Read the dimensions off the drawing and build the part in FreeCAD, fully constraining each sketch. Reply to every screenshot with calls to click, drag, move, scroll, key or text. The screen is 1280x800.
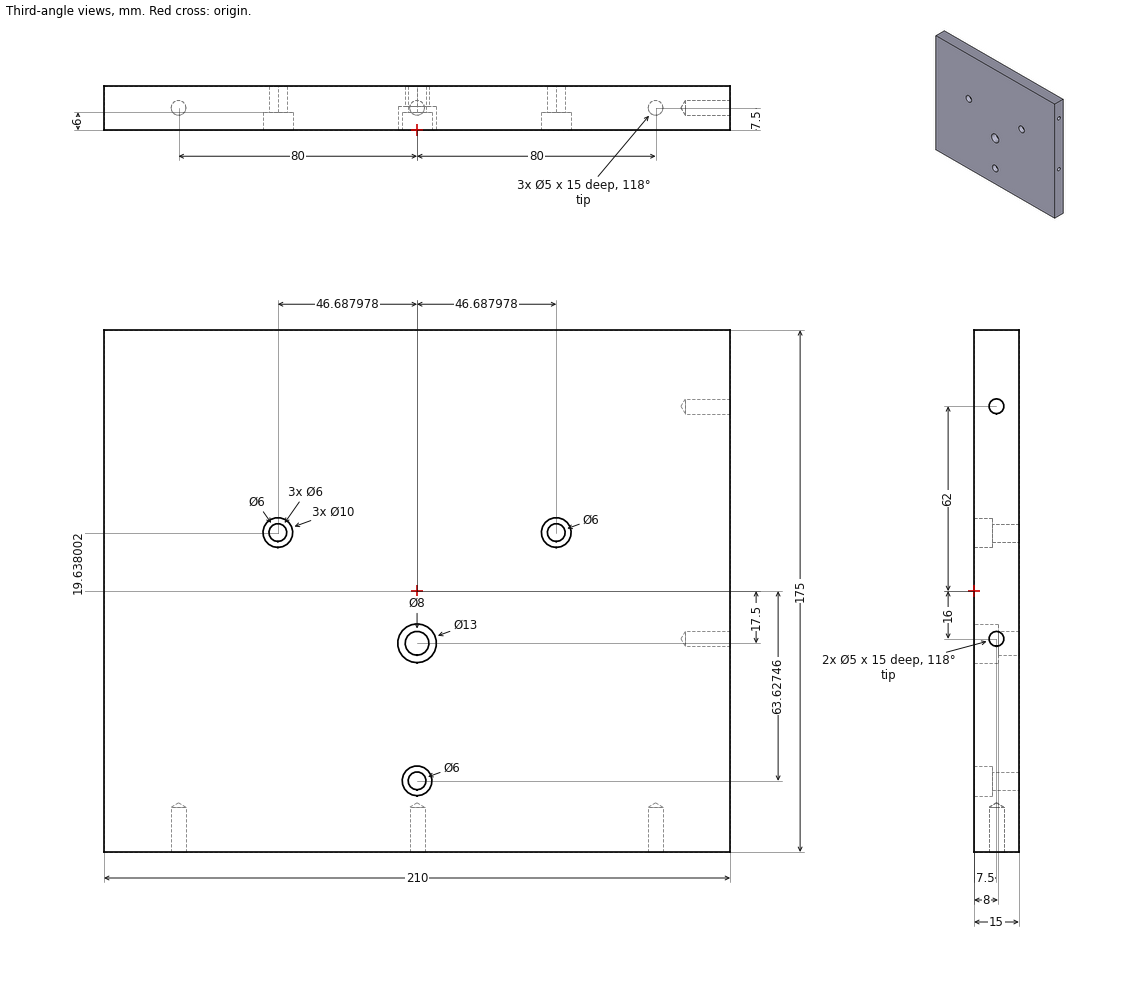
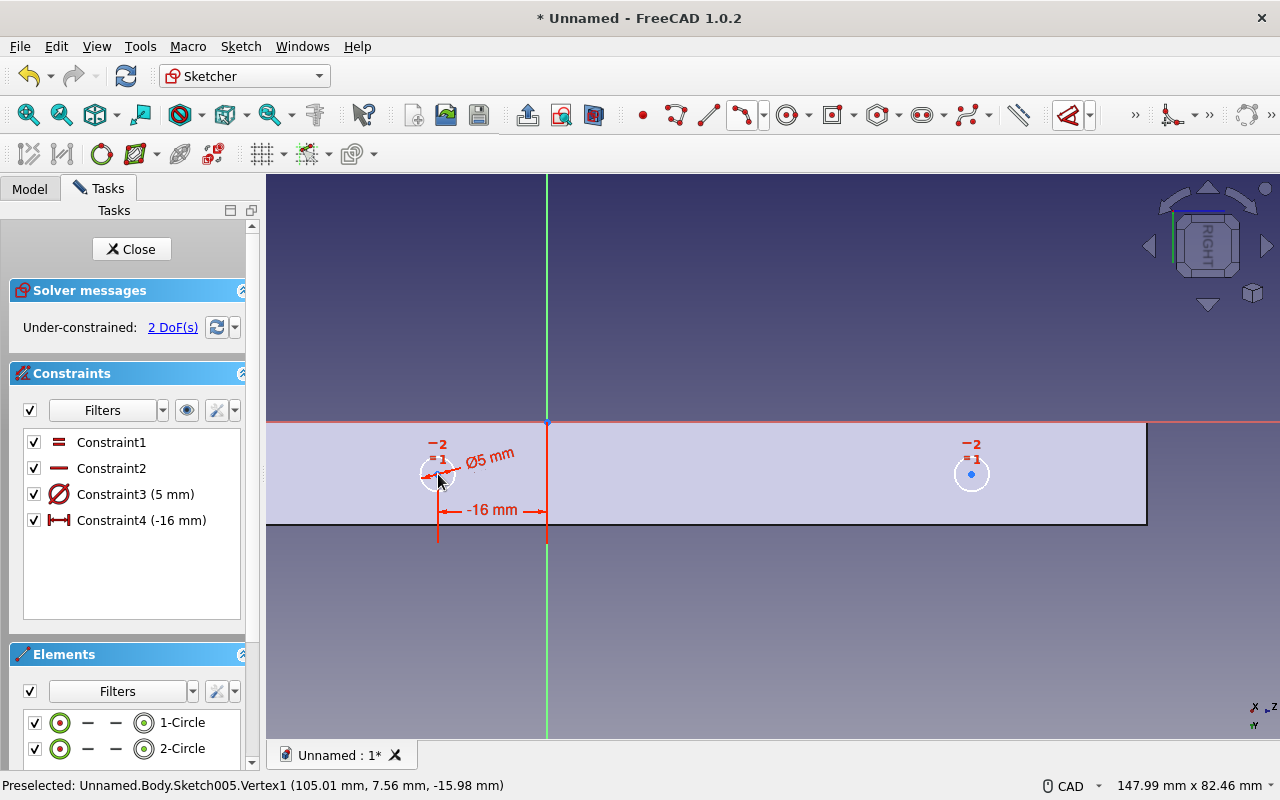
click(972, 474)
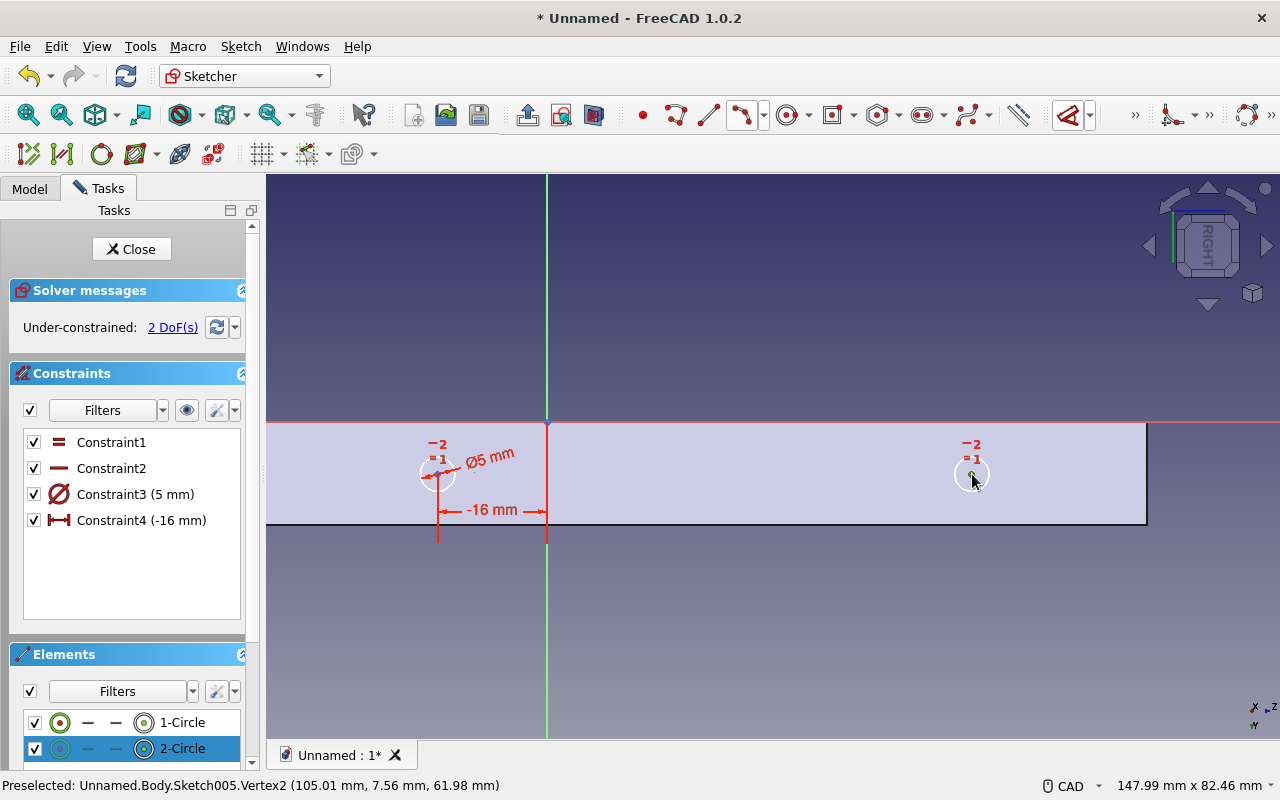
click(1090, 116)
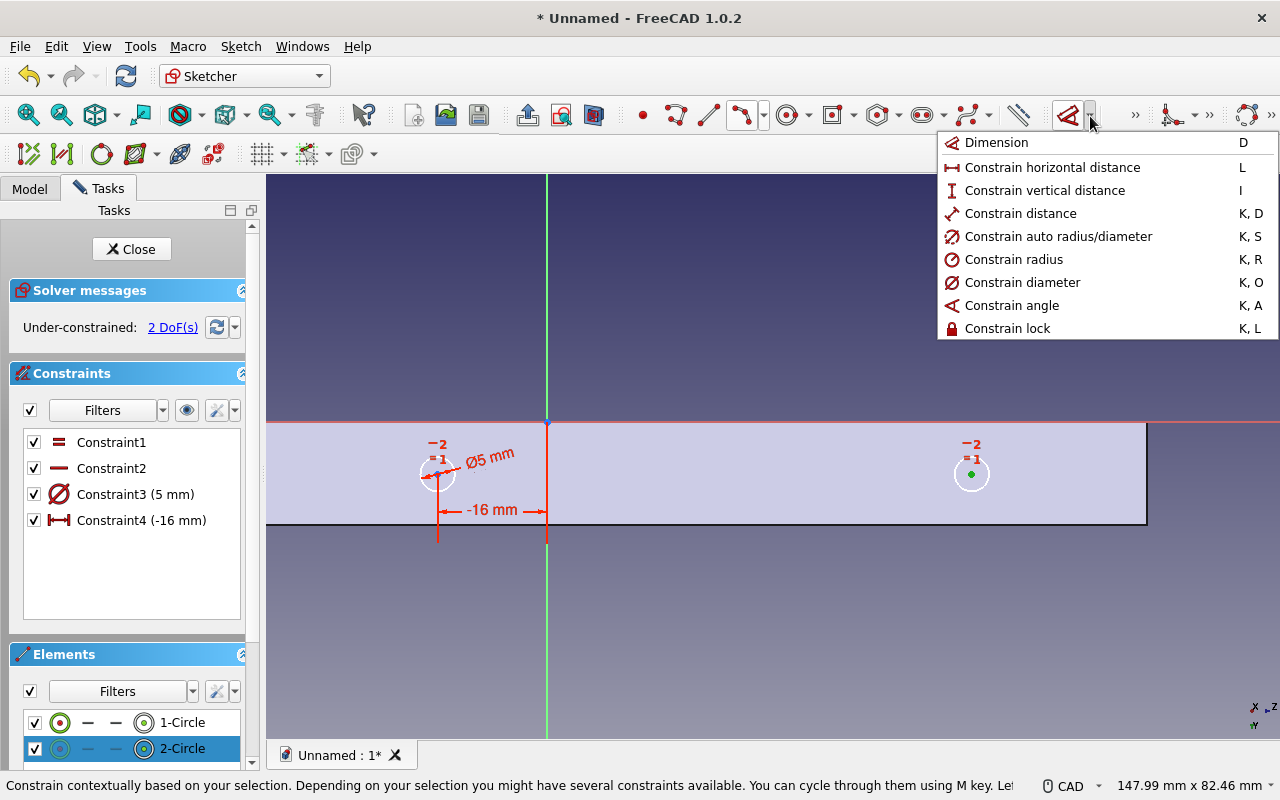
click(1108, 168)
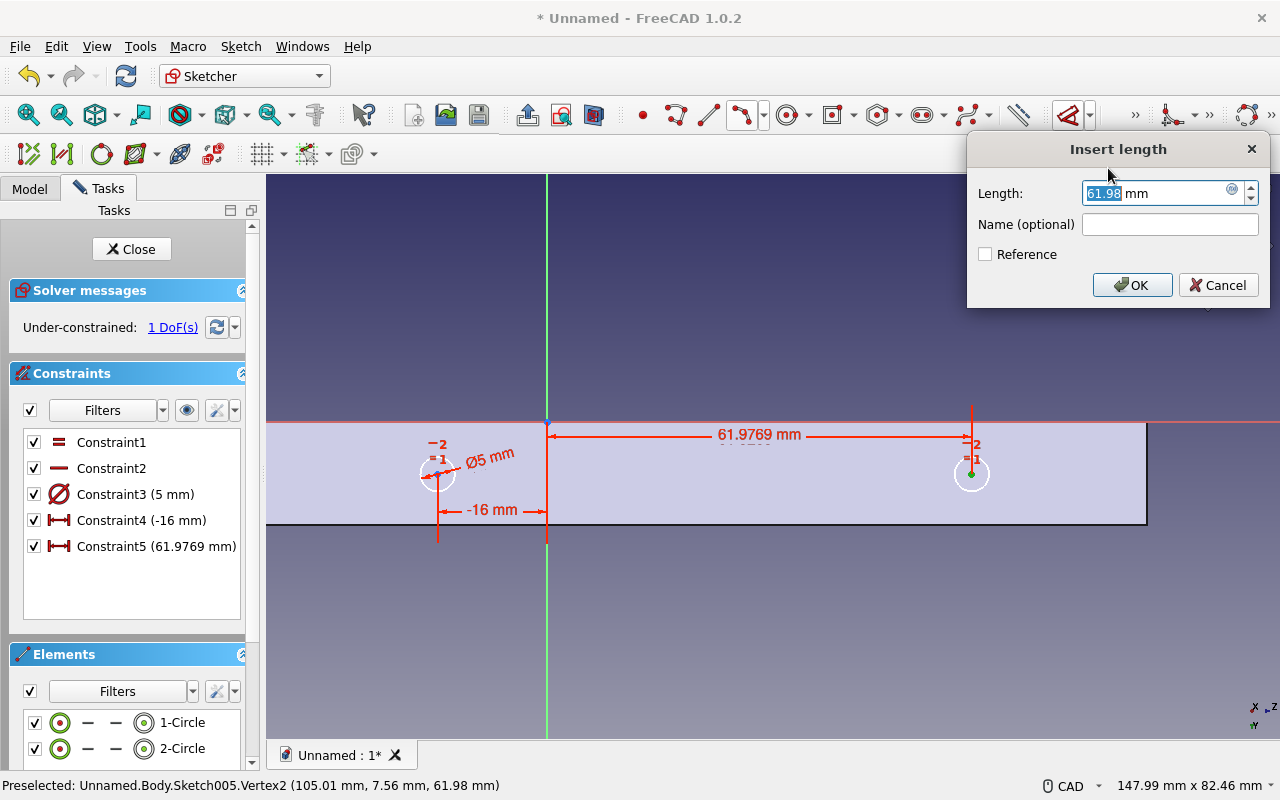
text(62)
key(Return)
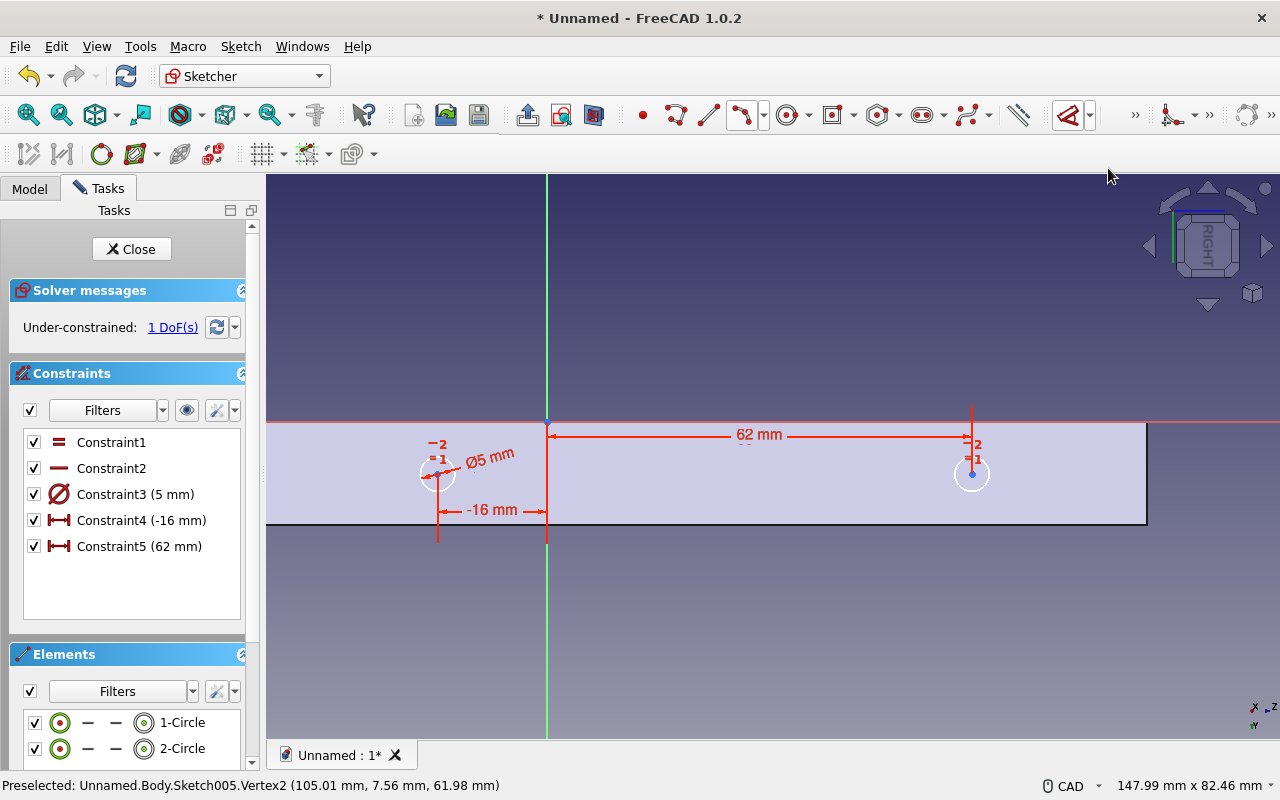
click(438, 474)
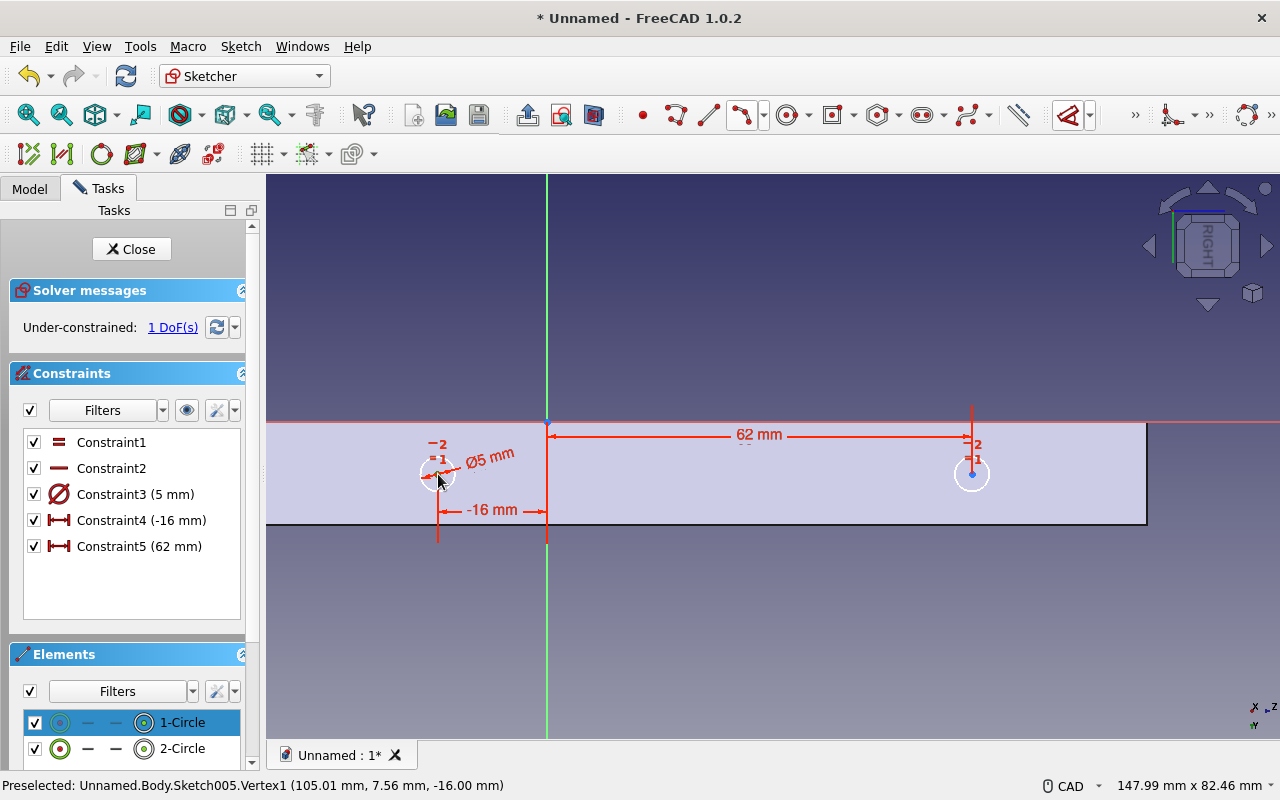
click(1090, 116)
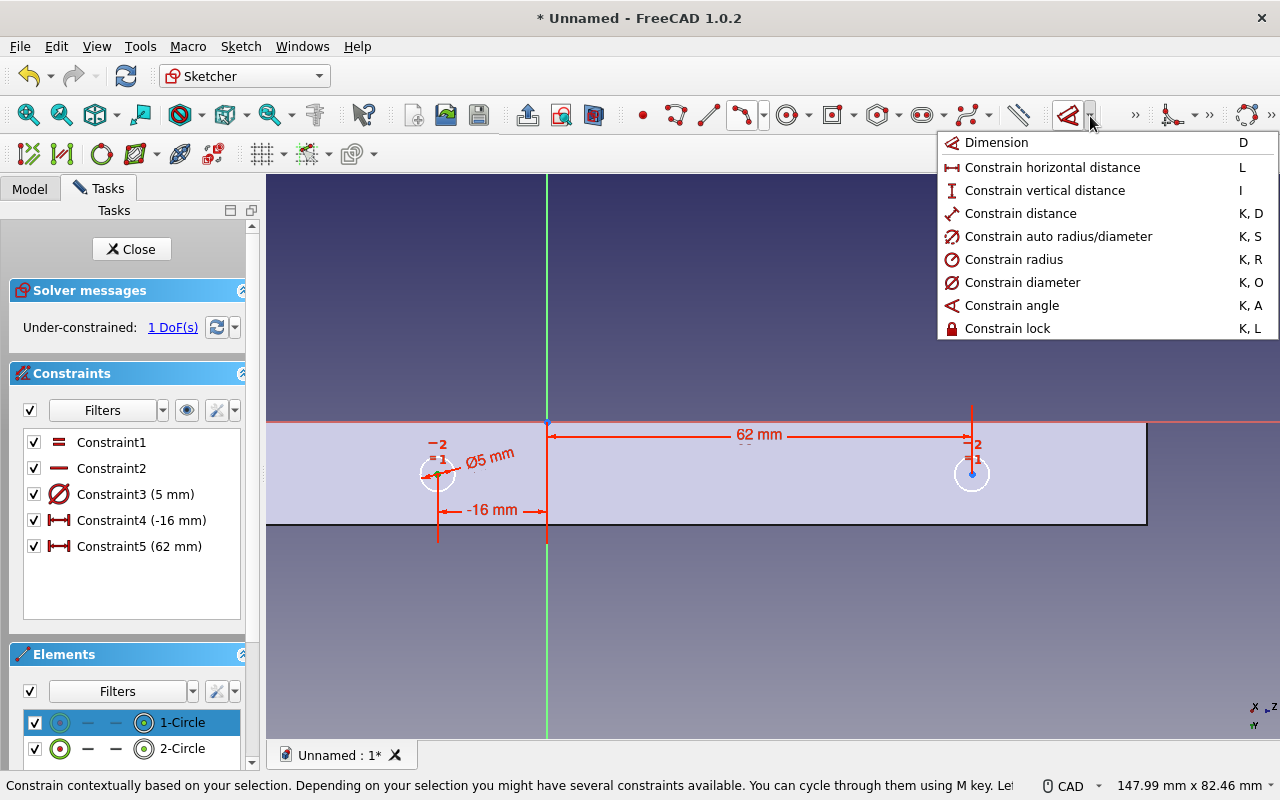
click(1108, 190)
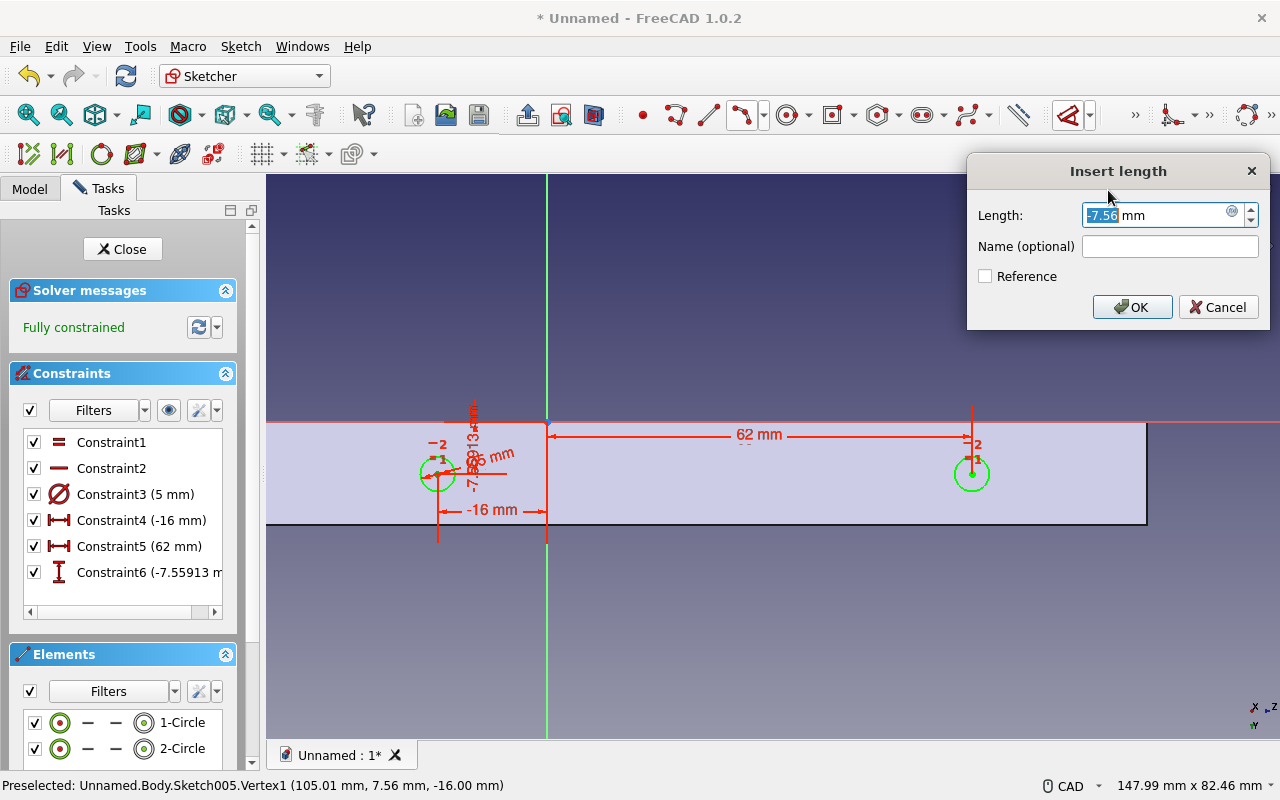
text(-7.5)
key(Return)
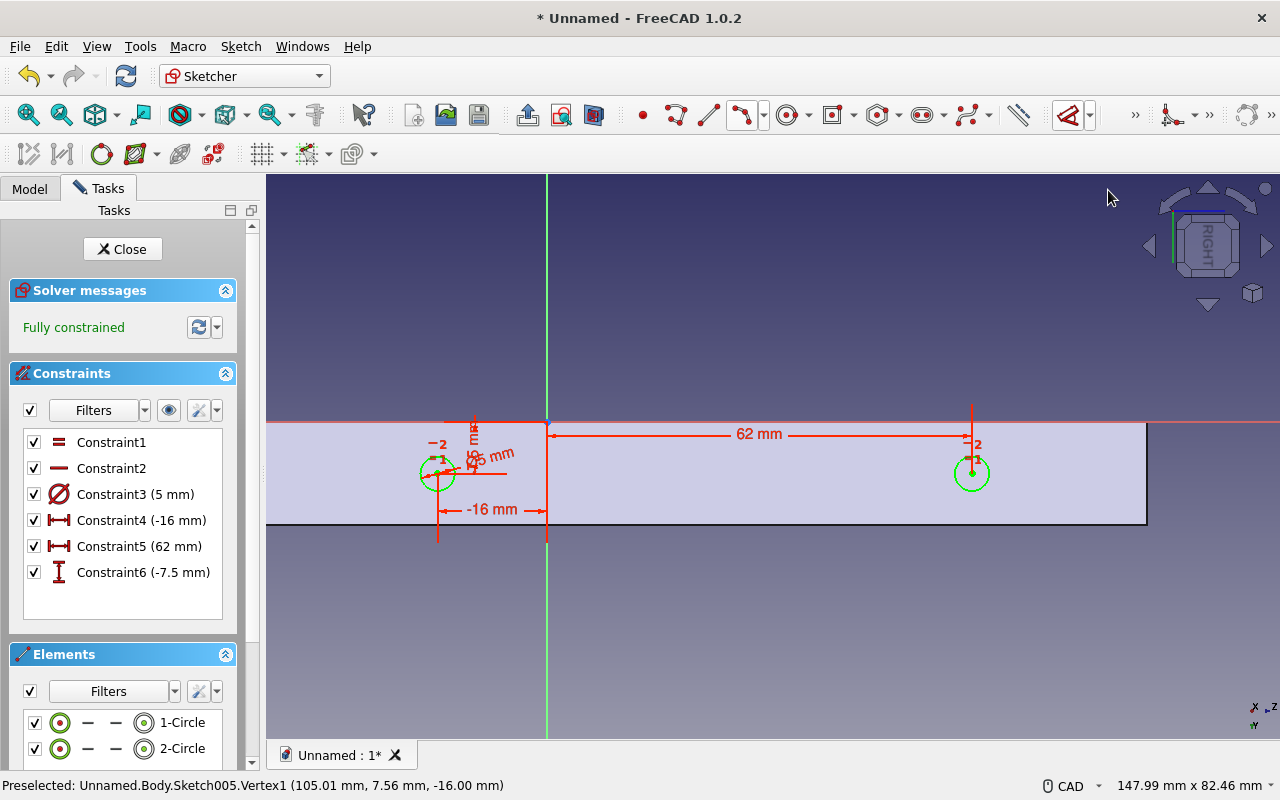
click(123, 249)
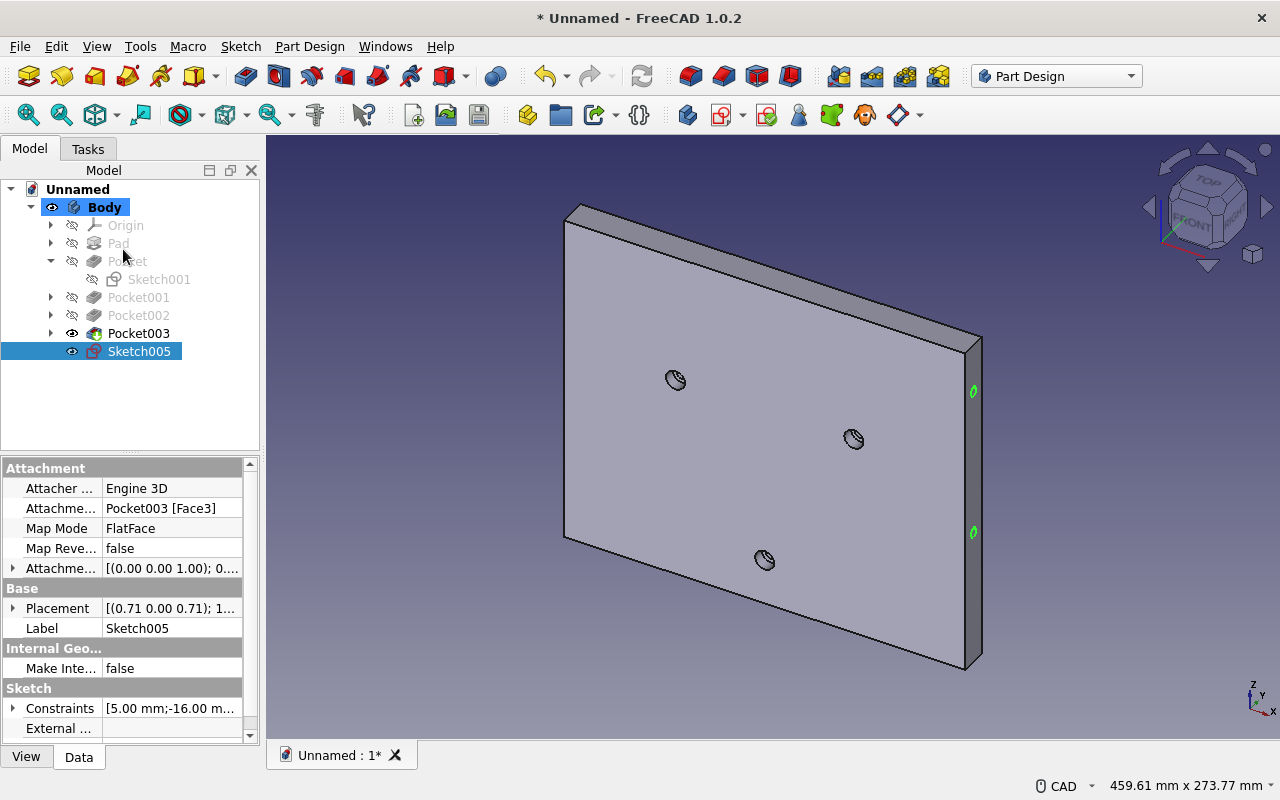
click(279, 76)